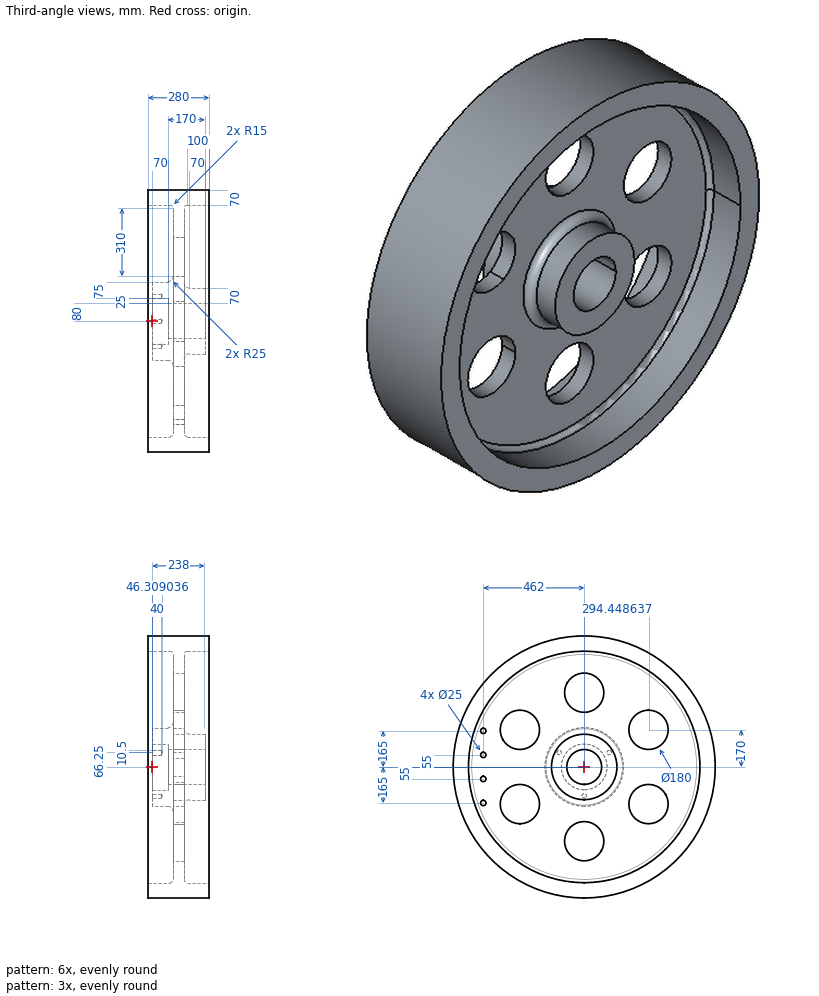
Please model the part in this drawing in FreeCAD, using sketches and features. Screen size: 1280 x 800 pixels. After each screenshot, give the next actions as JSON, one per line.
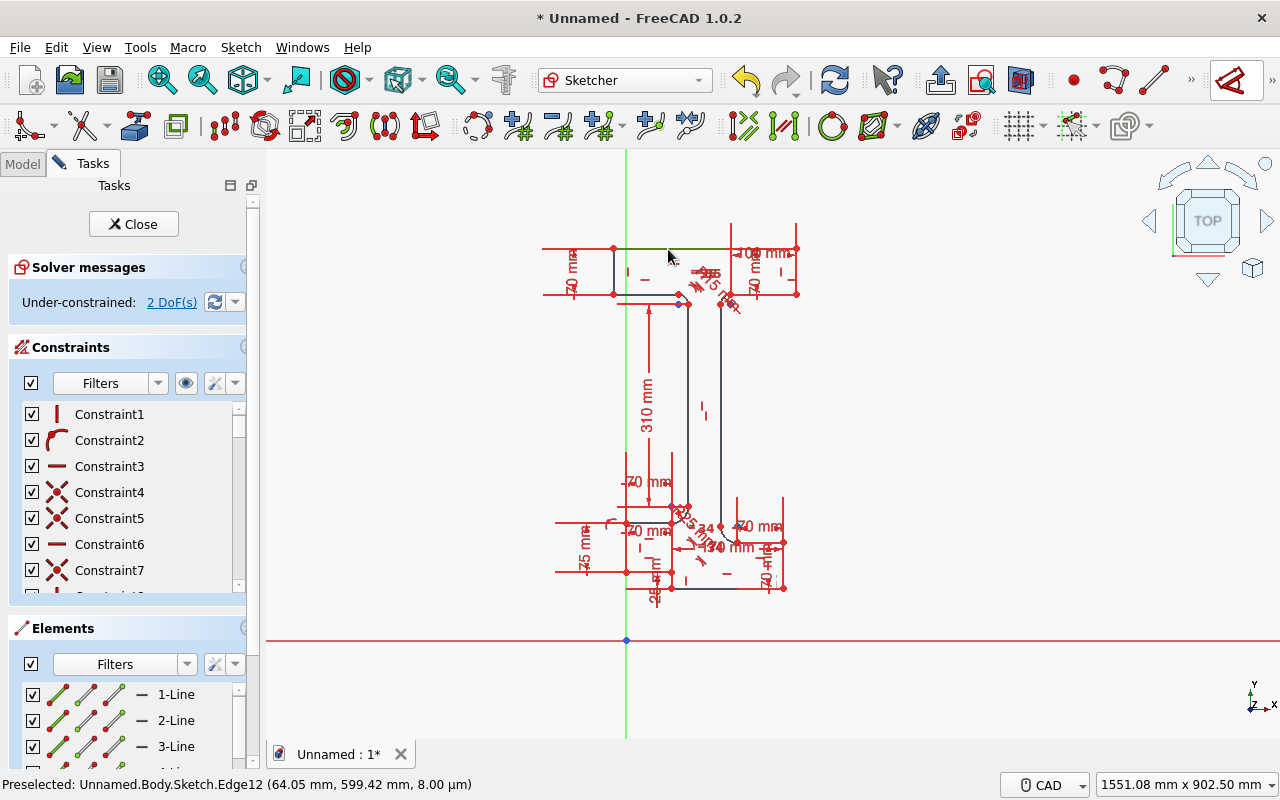
{"action": "left_click", "coordinate": [1258, 80]}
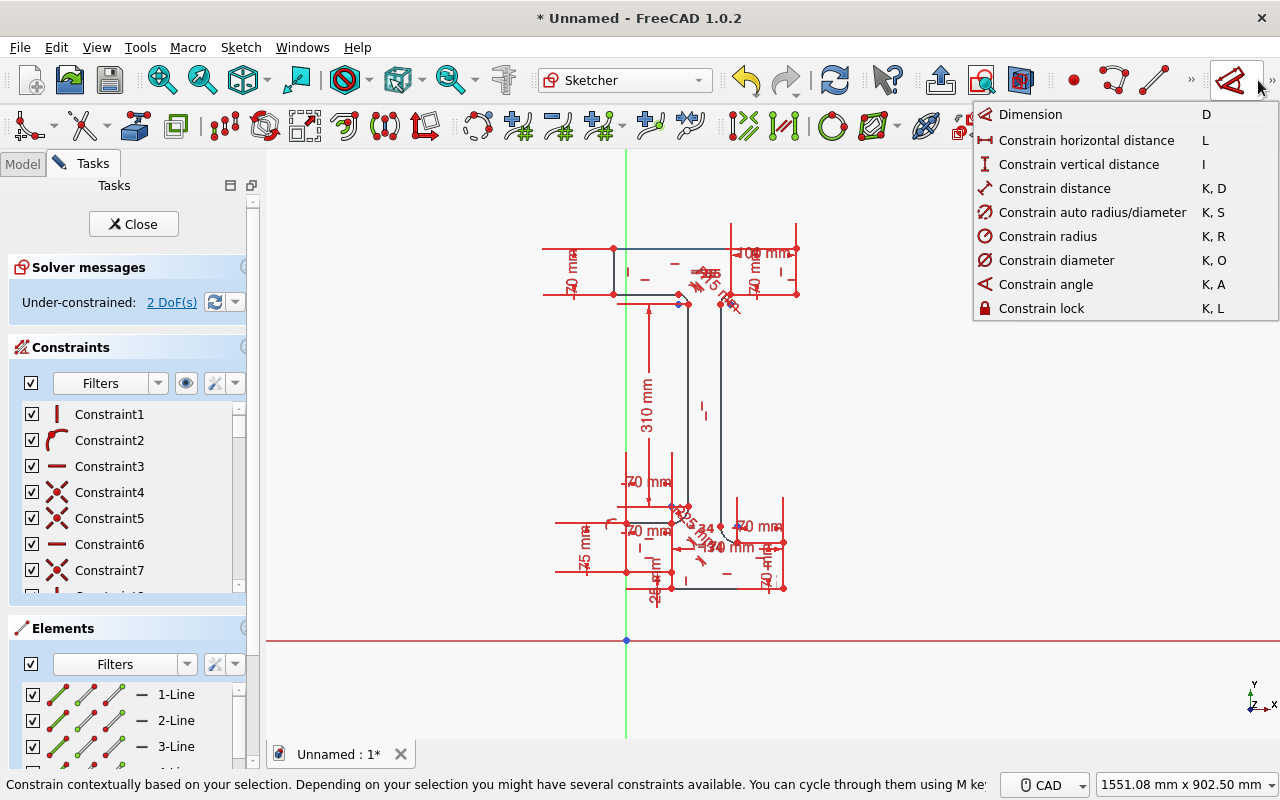
{"action": "left_click", "coordinate": [1126, 140]}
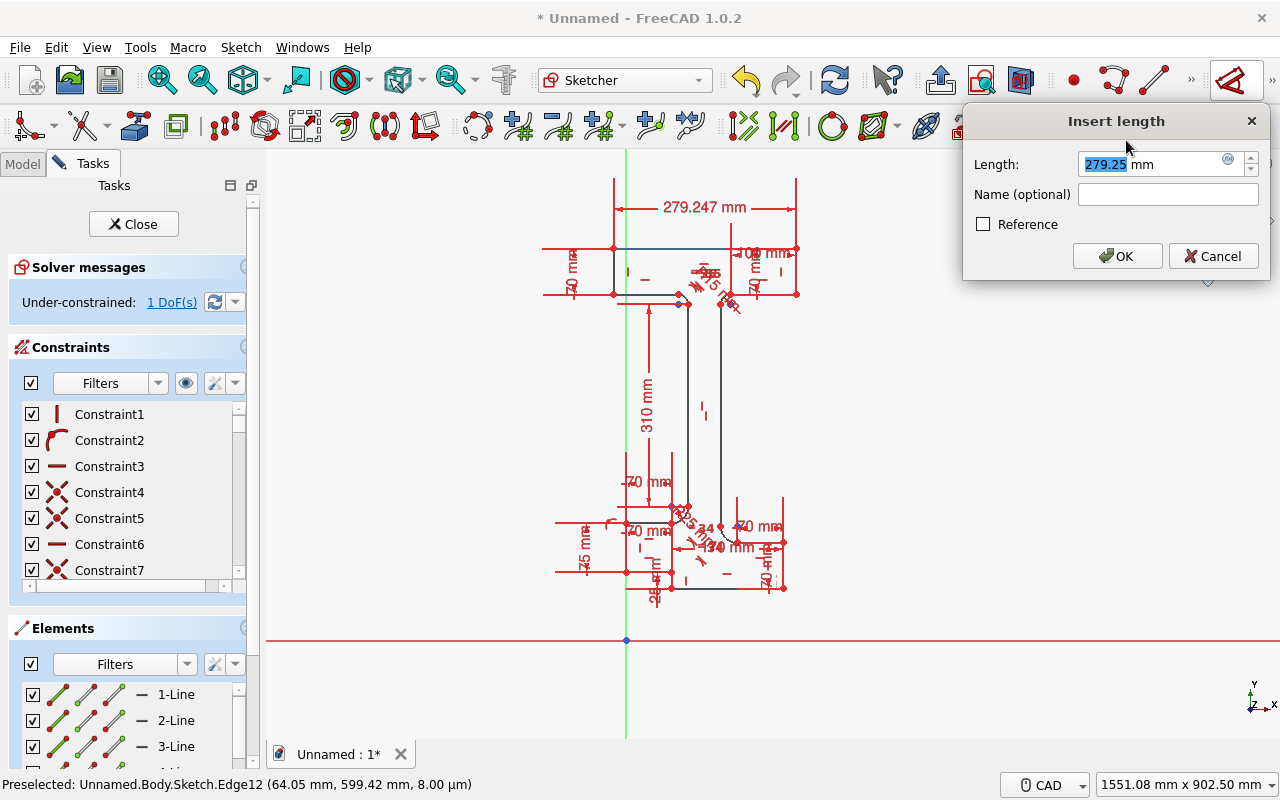
{"action": "type", "text": "280"}
{"action": "key", "text": "Return"}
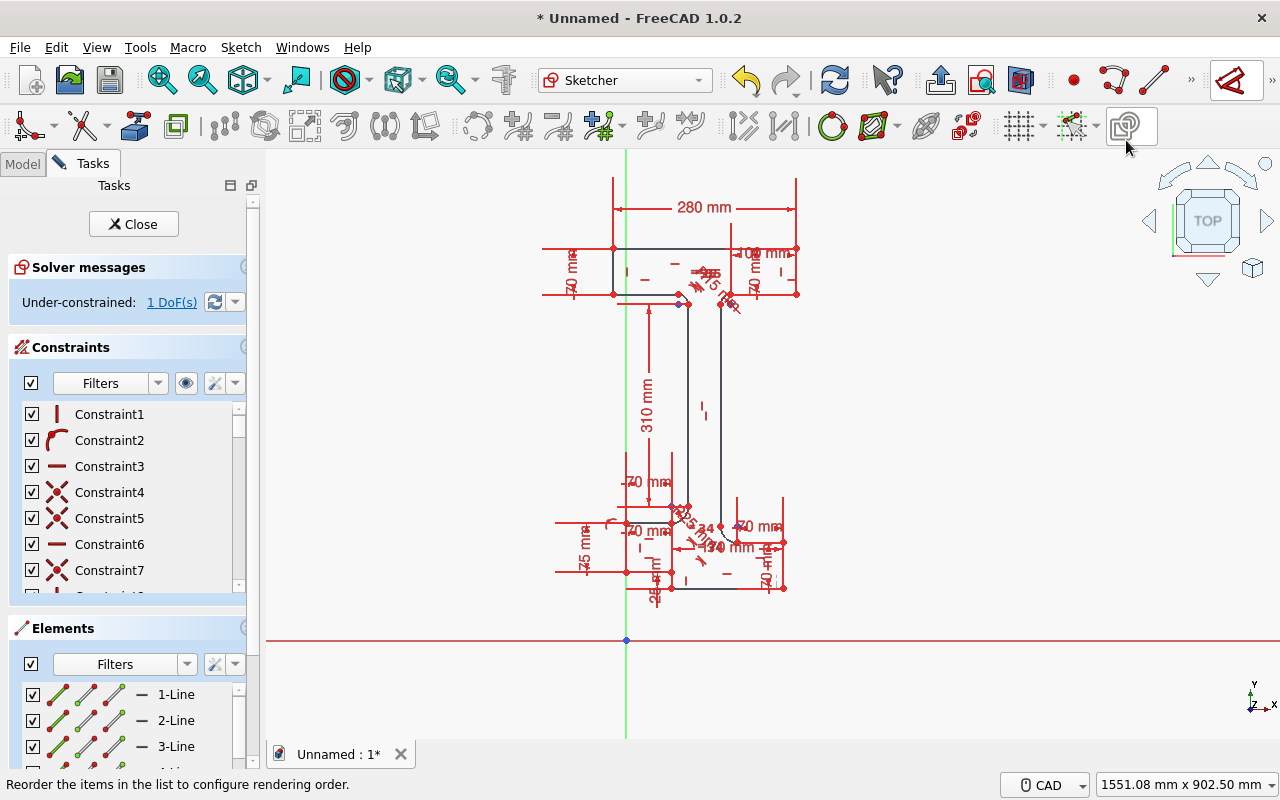
{"action": "left_click", "coordinate": [672, 589]}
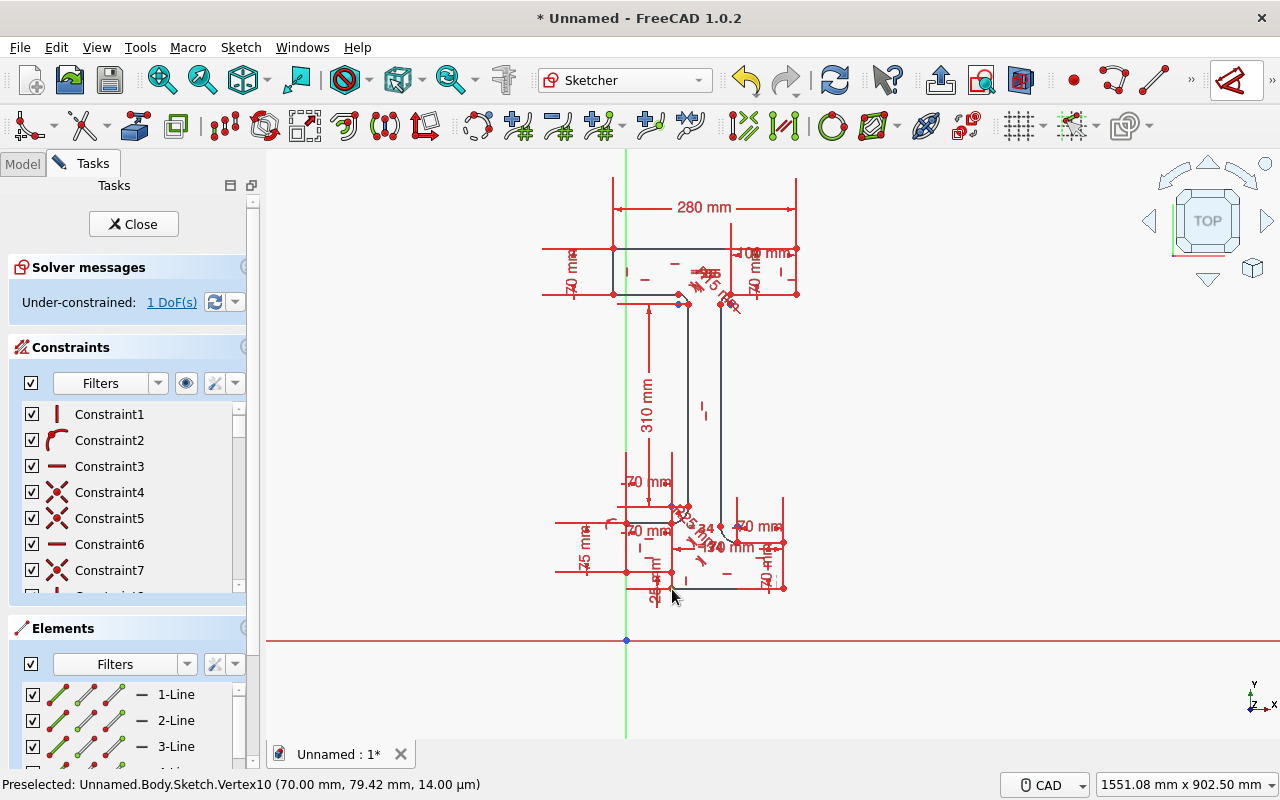
{"action": "left_click", "coordinate": [1258, 80]}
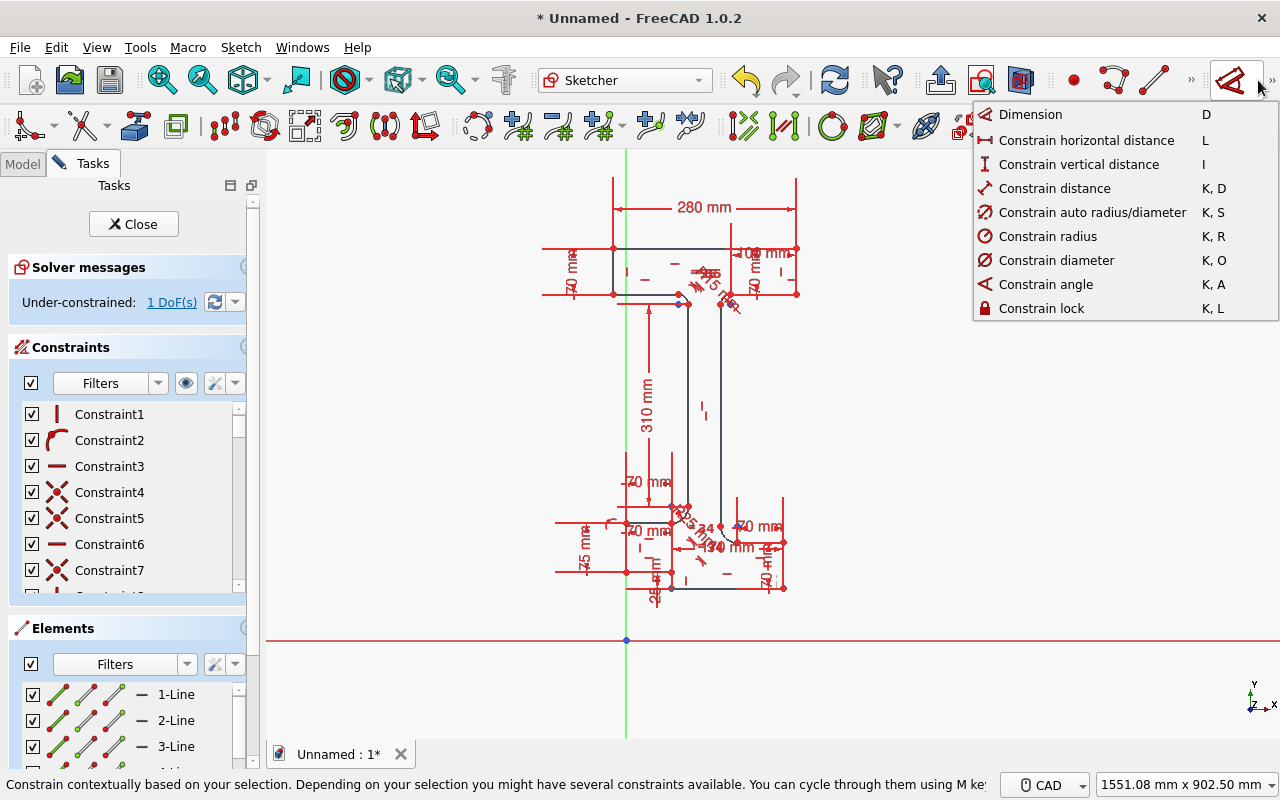
{"action": "left_click", "coordinate": [1126, 164]}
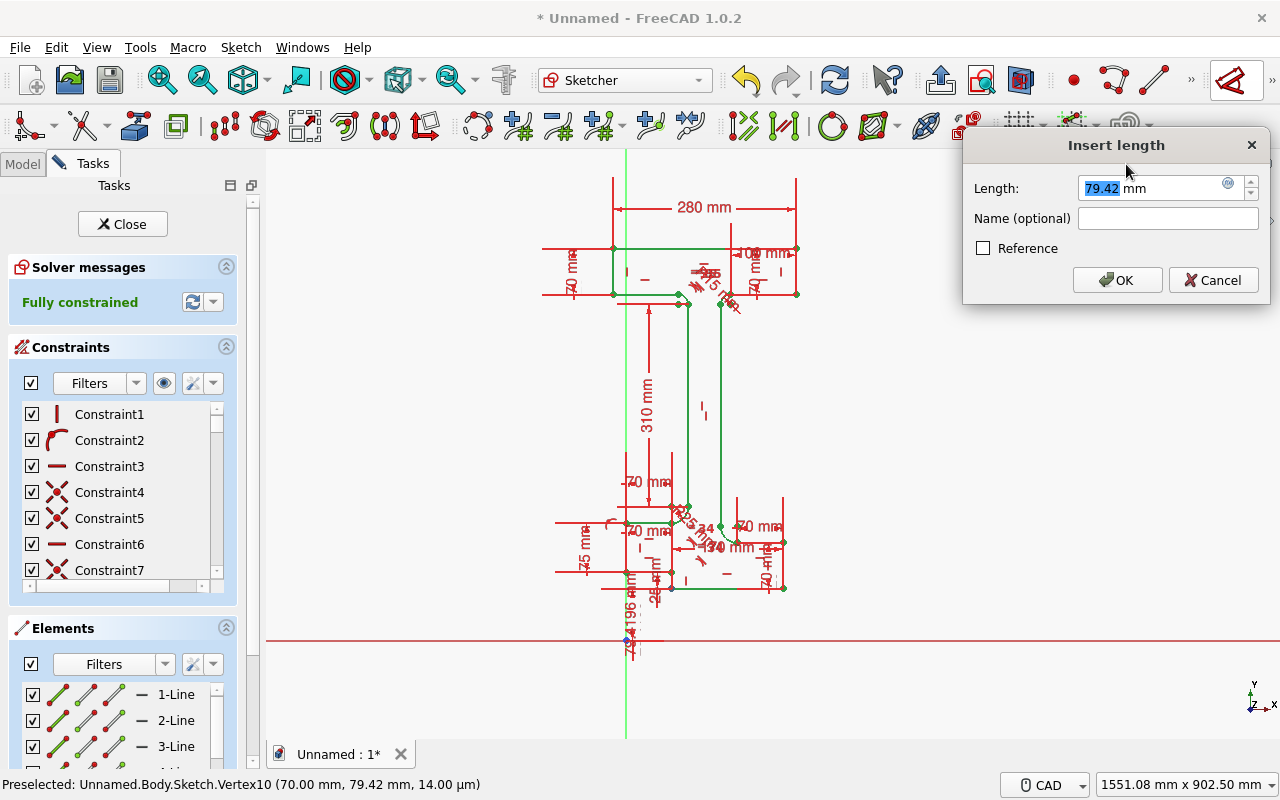
{"action": "type", "text": "80"}
{"action": "key", "text": "Return"}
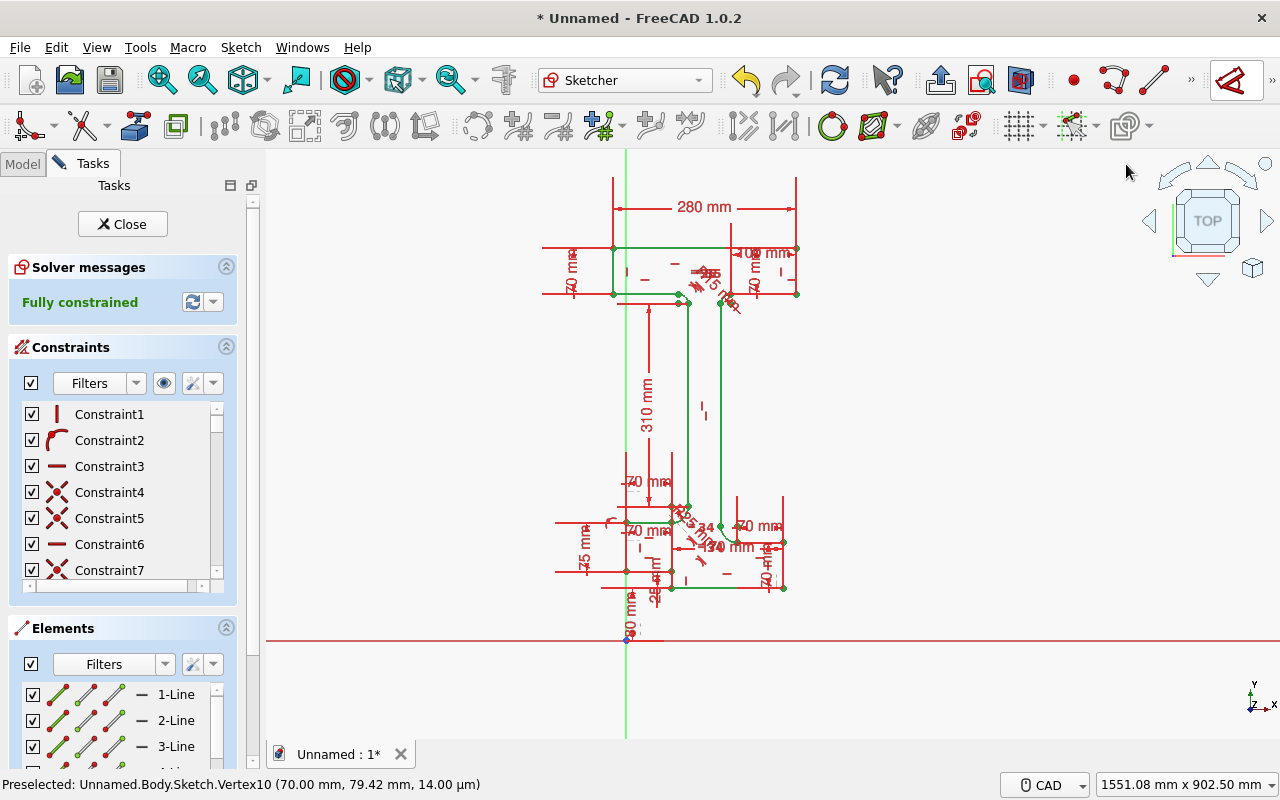
{"action": "left_click", "coordinate": [123, 224]}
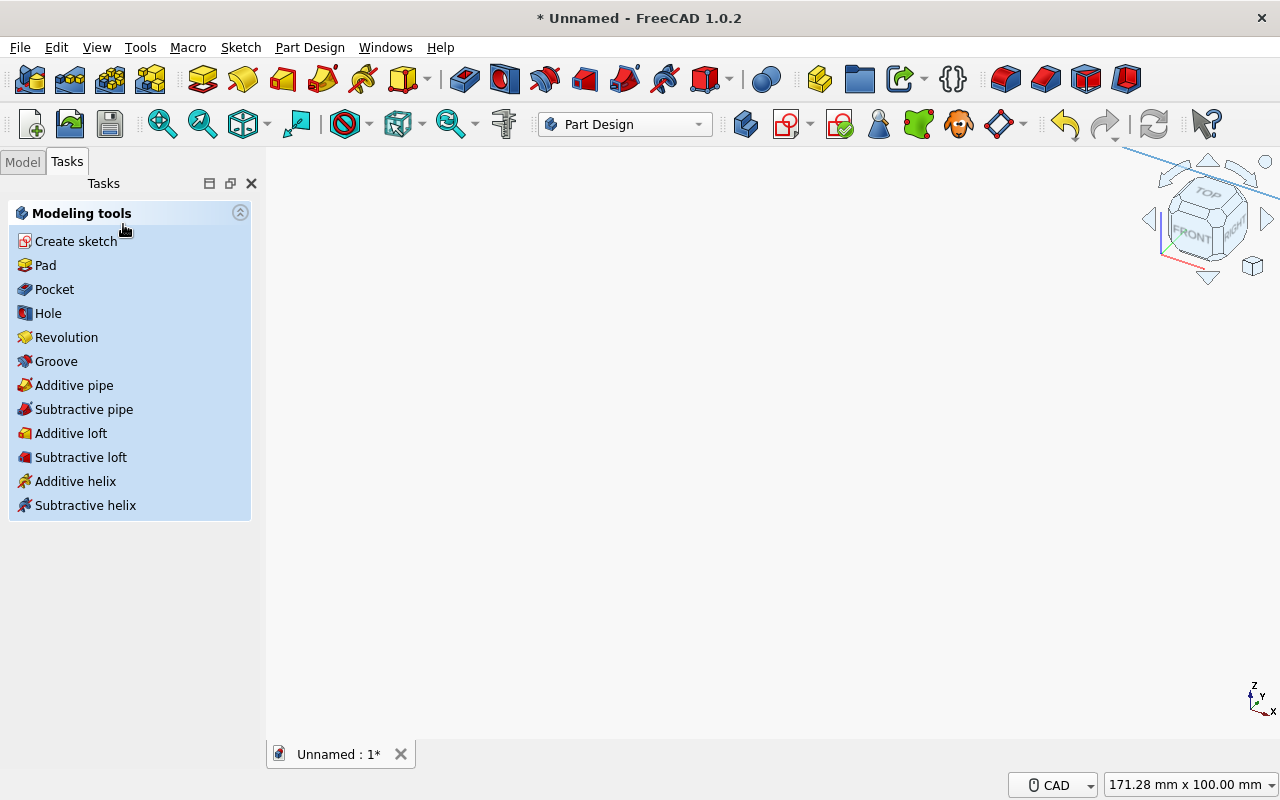
{"action": "left_click", "coordinate": [244, 80]}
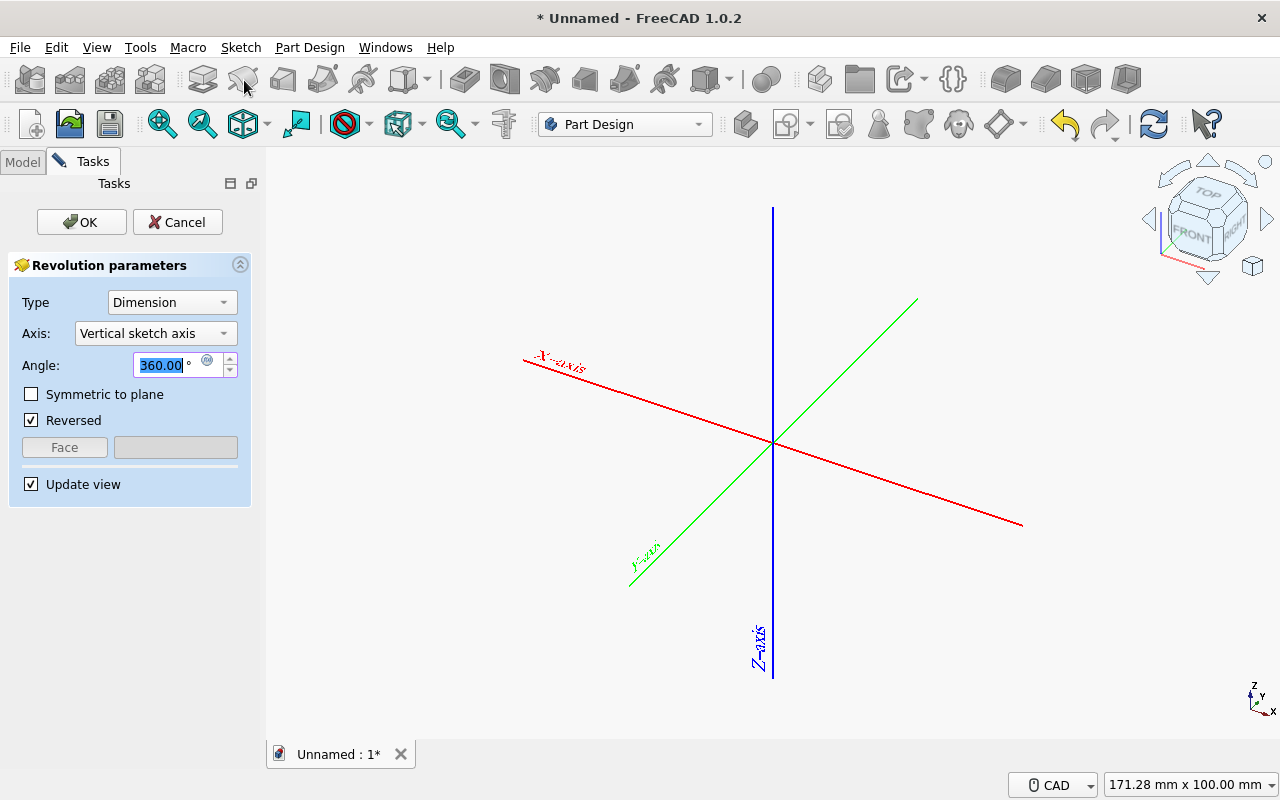
{"action": "left_click", "coordinate": [156, 334]}